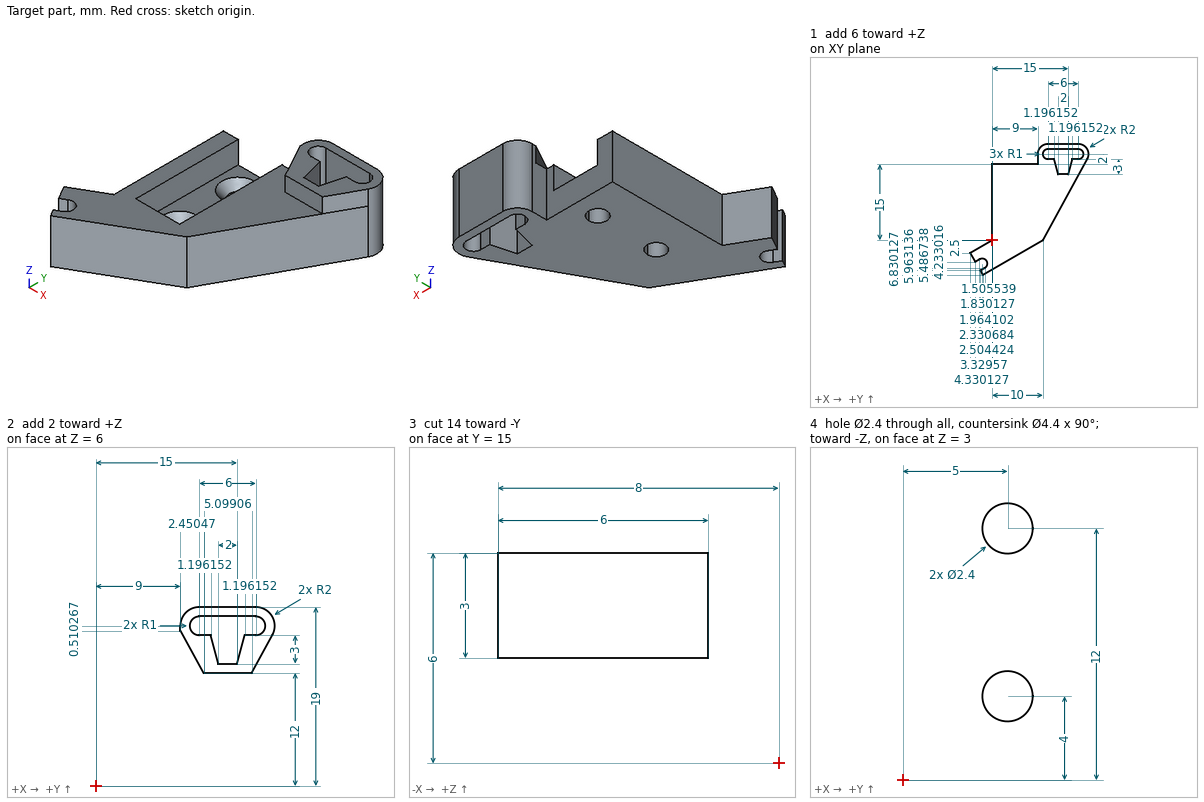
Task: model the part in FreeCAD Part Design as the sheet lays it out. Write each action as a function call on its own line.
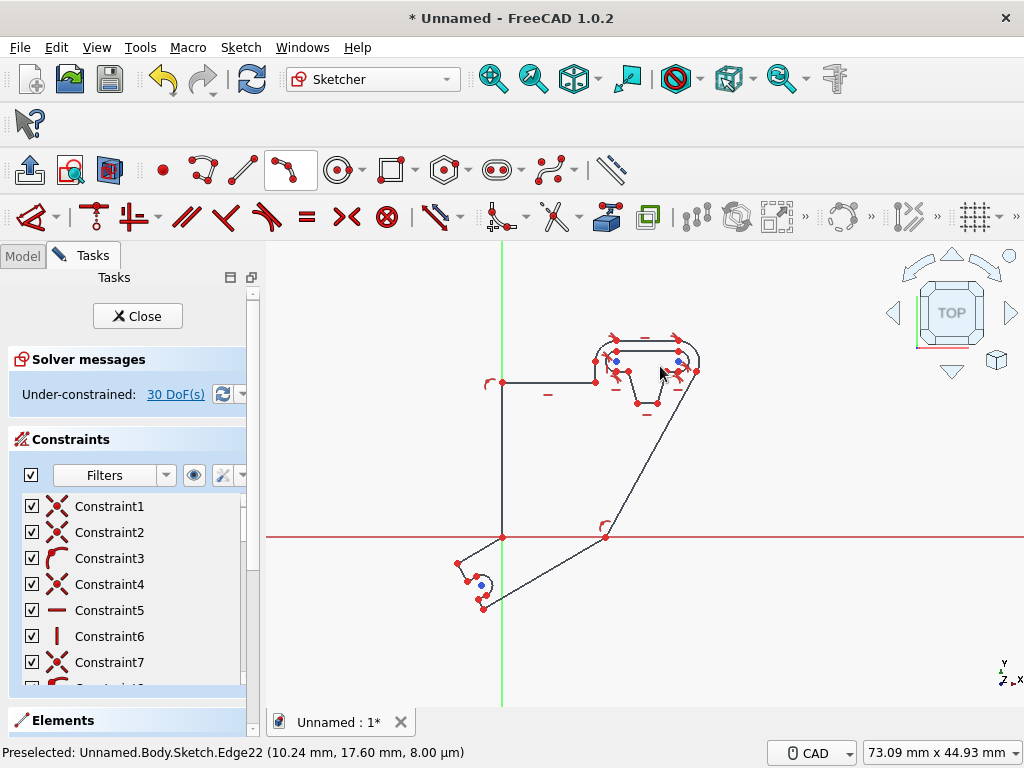
scroll(699, 359, up, 2)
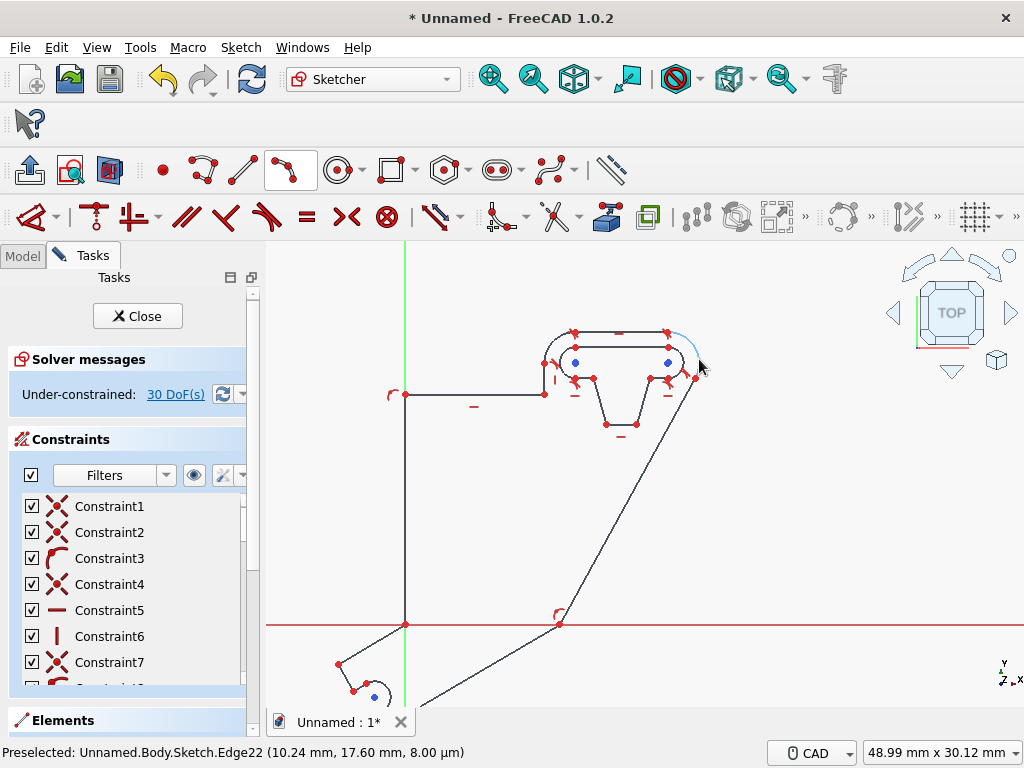
click(699, 360)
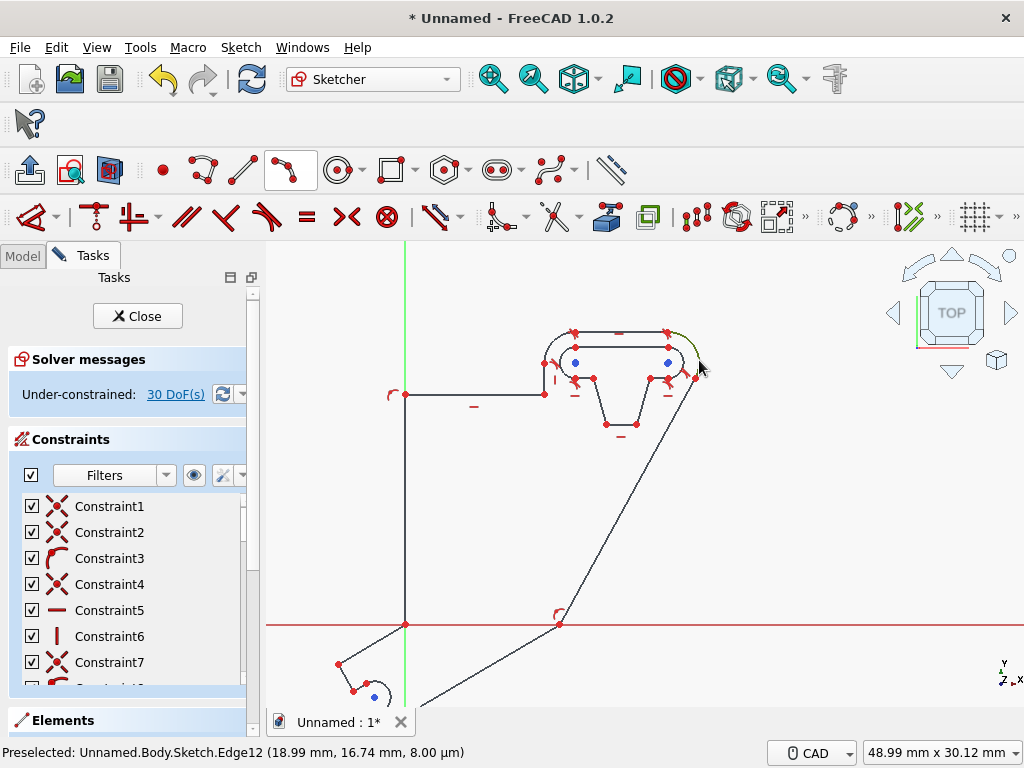
click(681, 354)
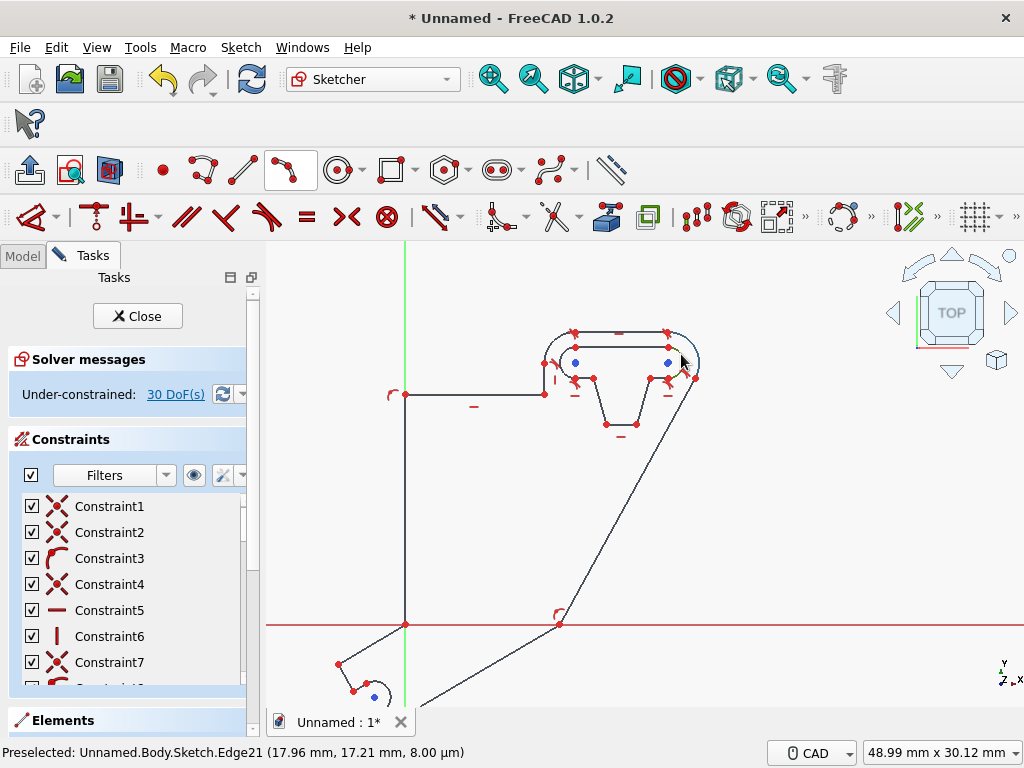
click(94, 218)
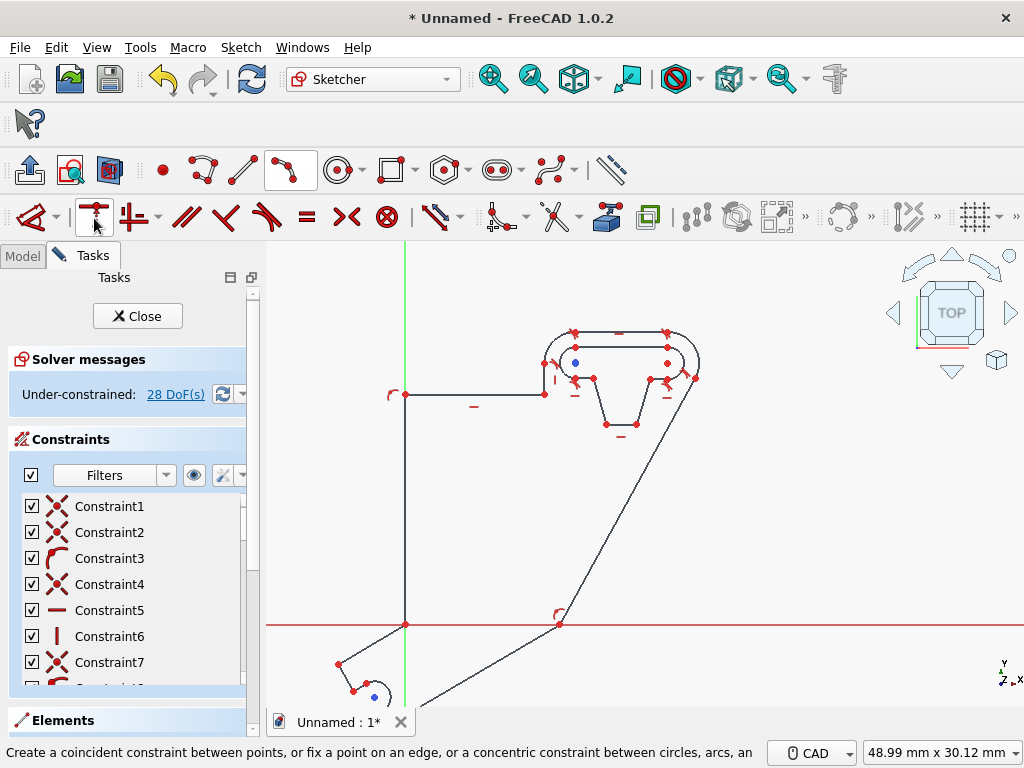
click(561, 335)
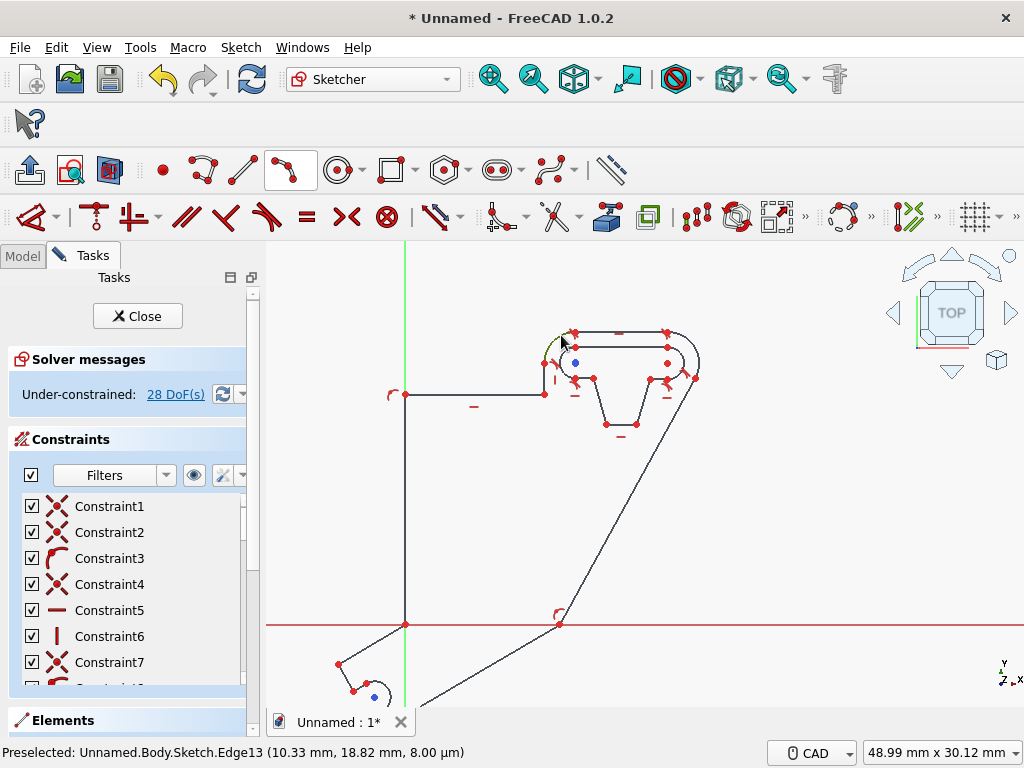
click(563, 354)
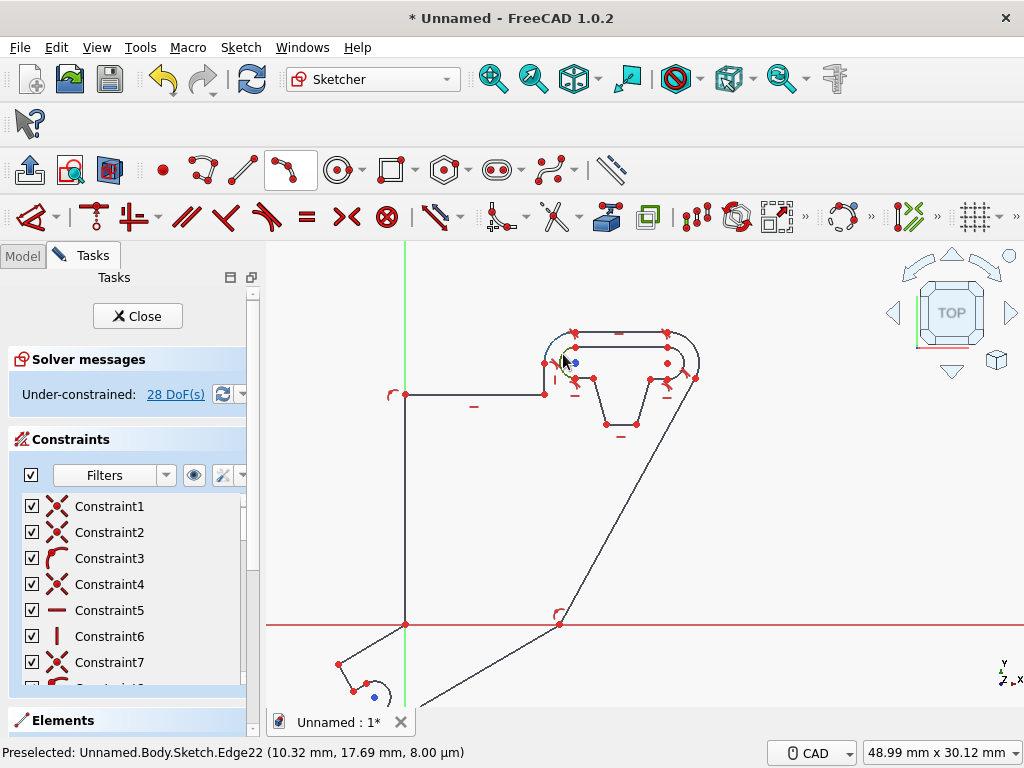
key(c)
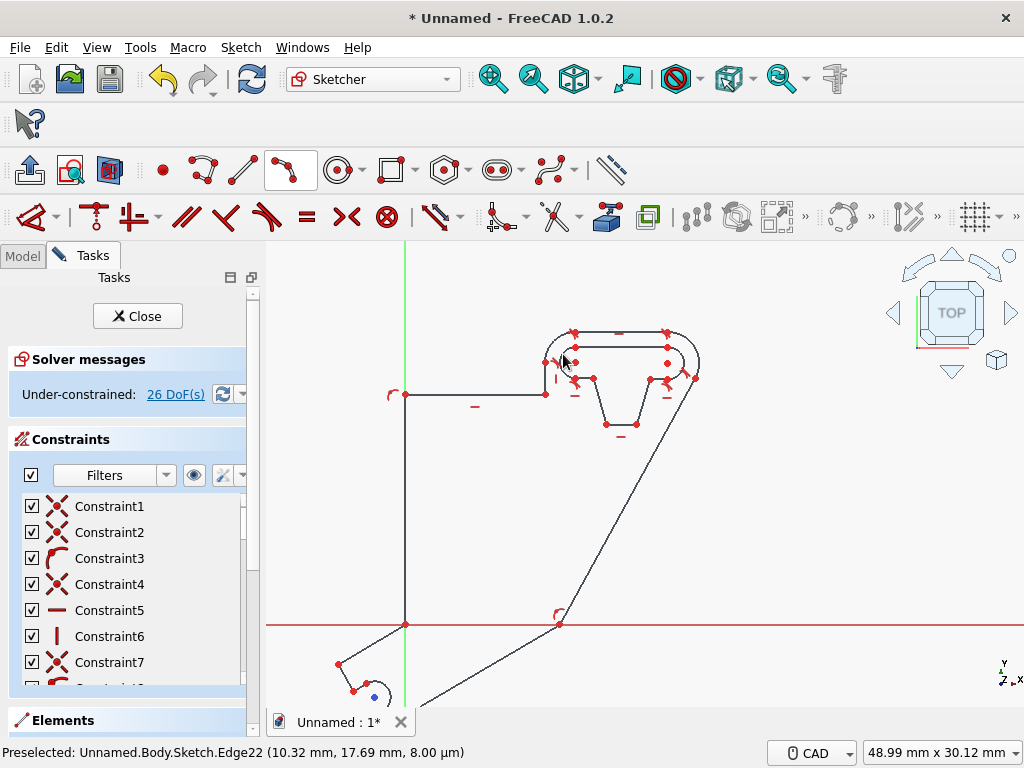
click(699, 360)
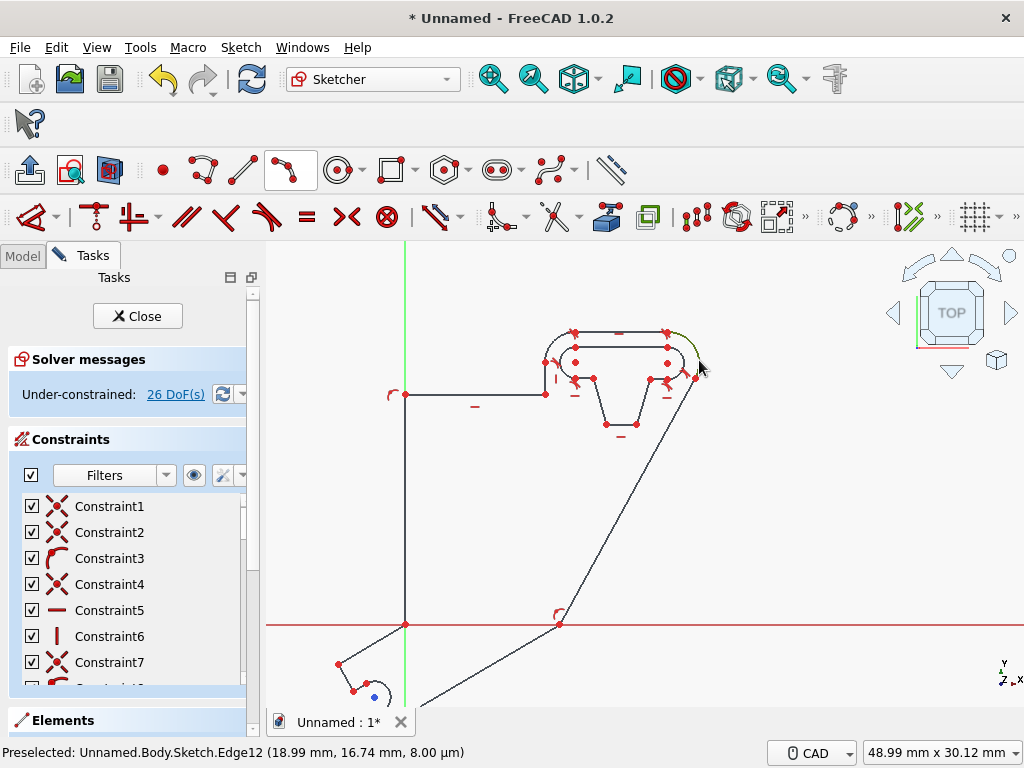
click(562, 335)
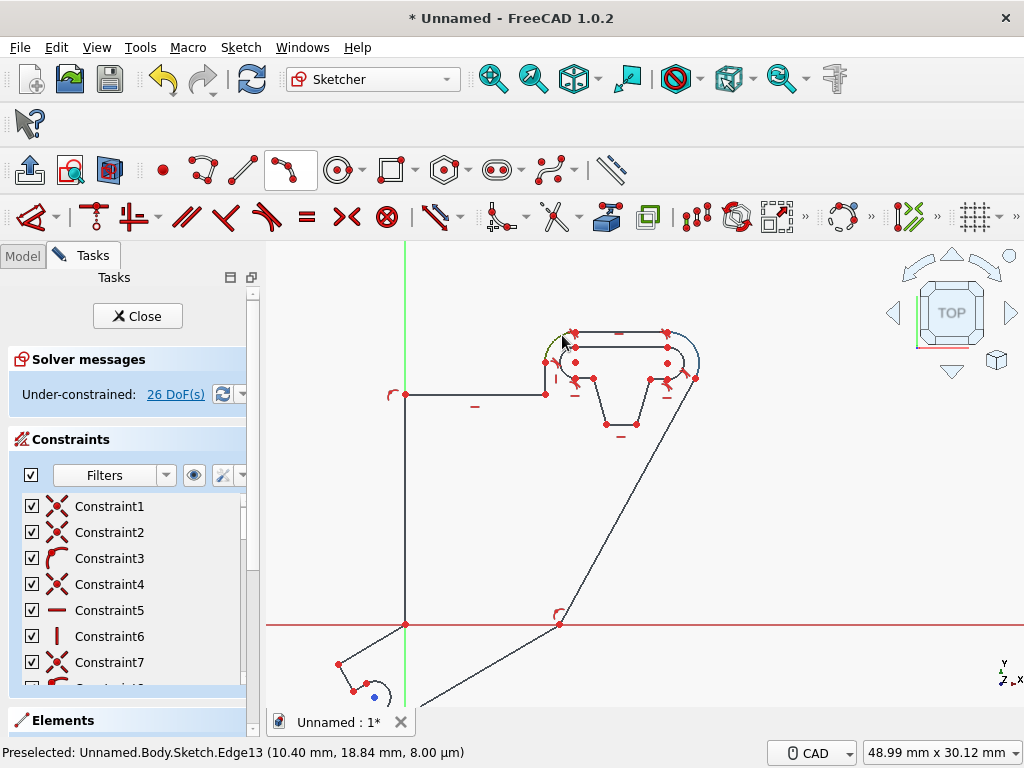
key(e)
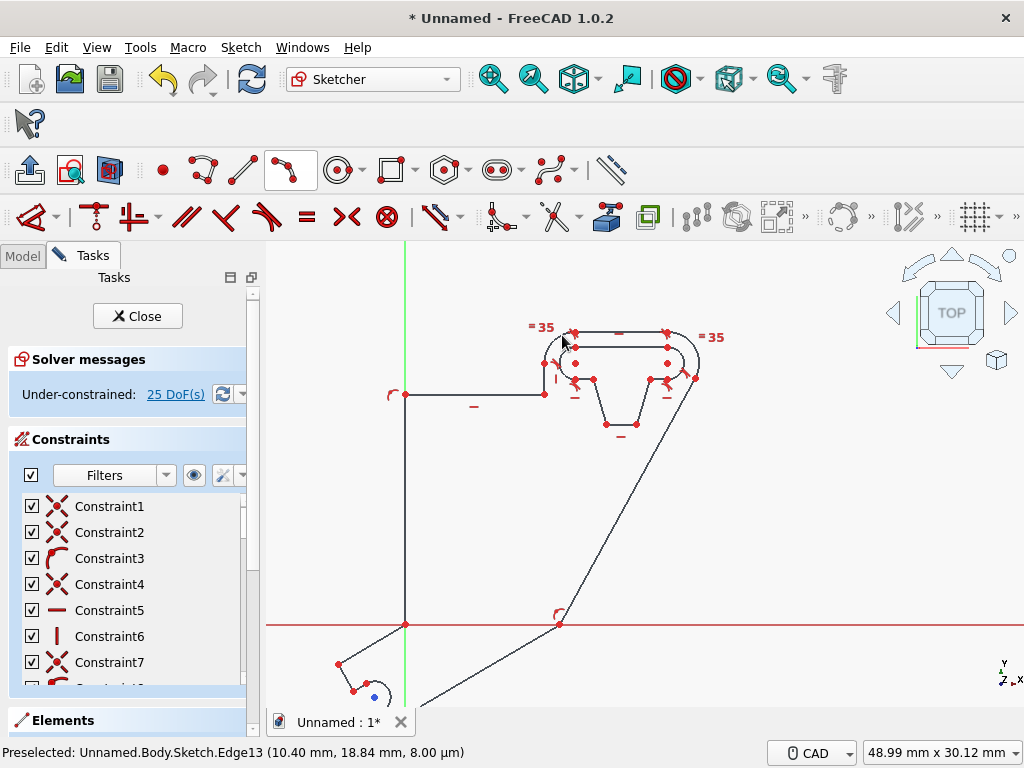
scroll(698, 358, down, 2)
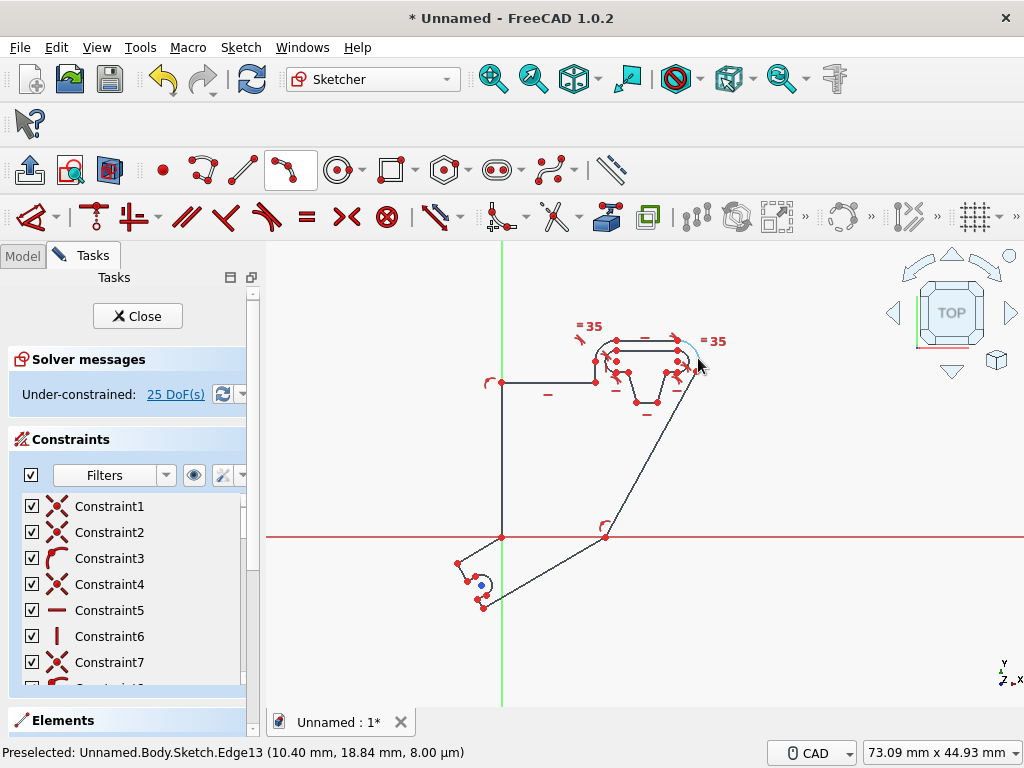
scroll(492, 587, up, 2)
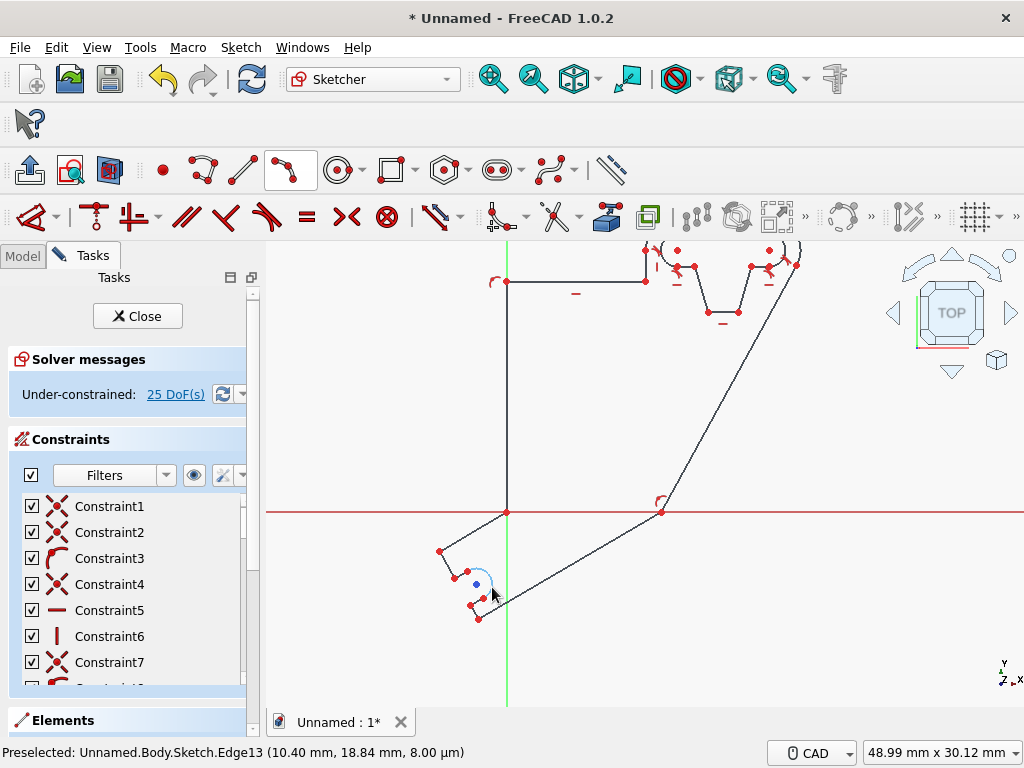
click(492, 587)